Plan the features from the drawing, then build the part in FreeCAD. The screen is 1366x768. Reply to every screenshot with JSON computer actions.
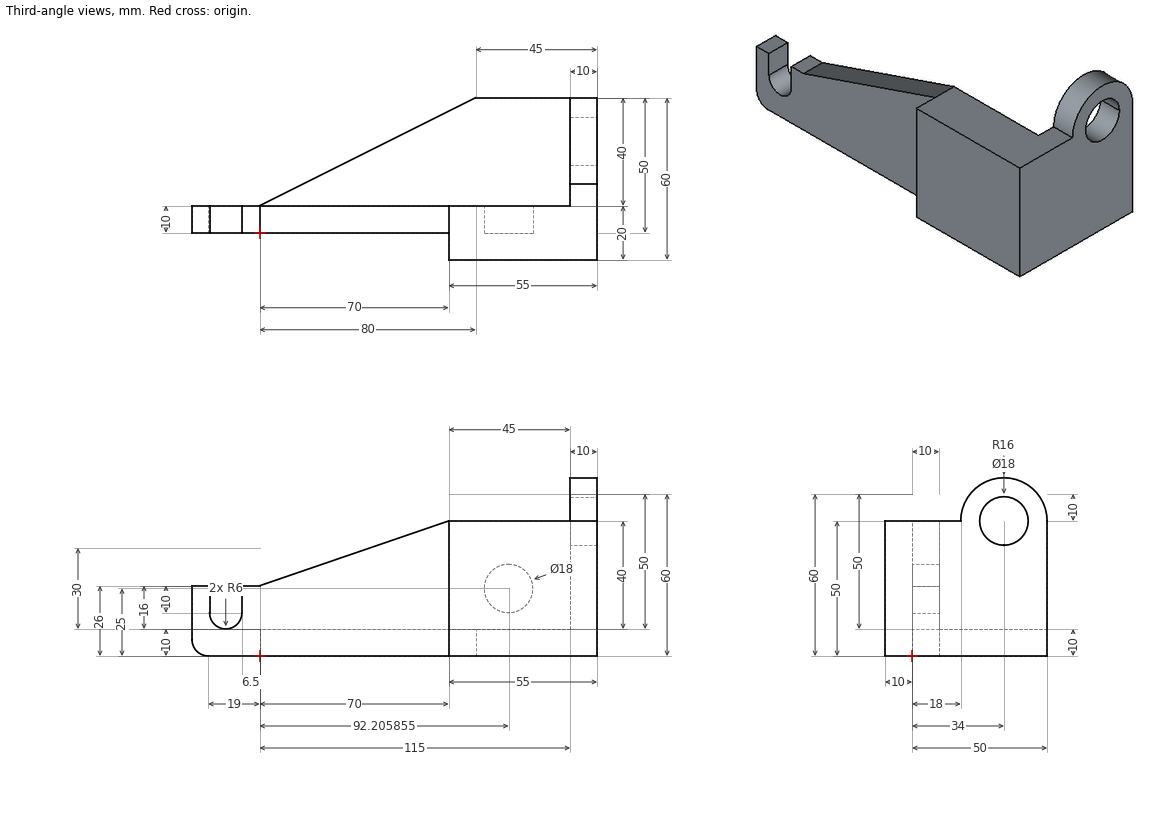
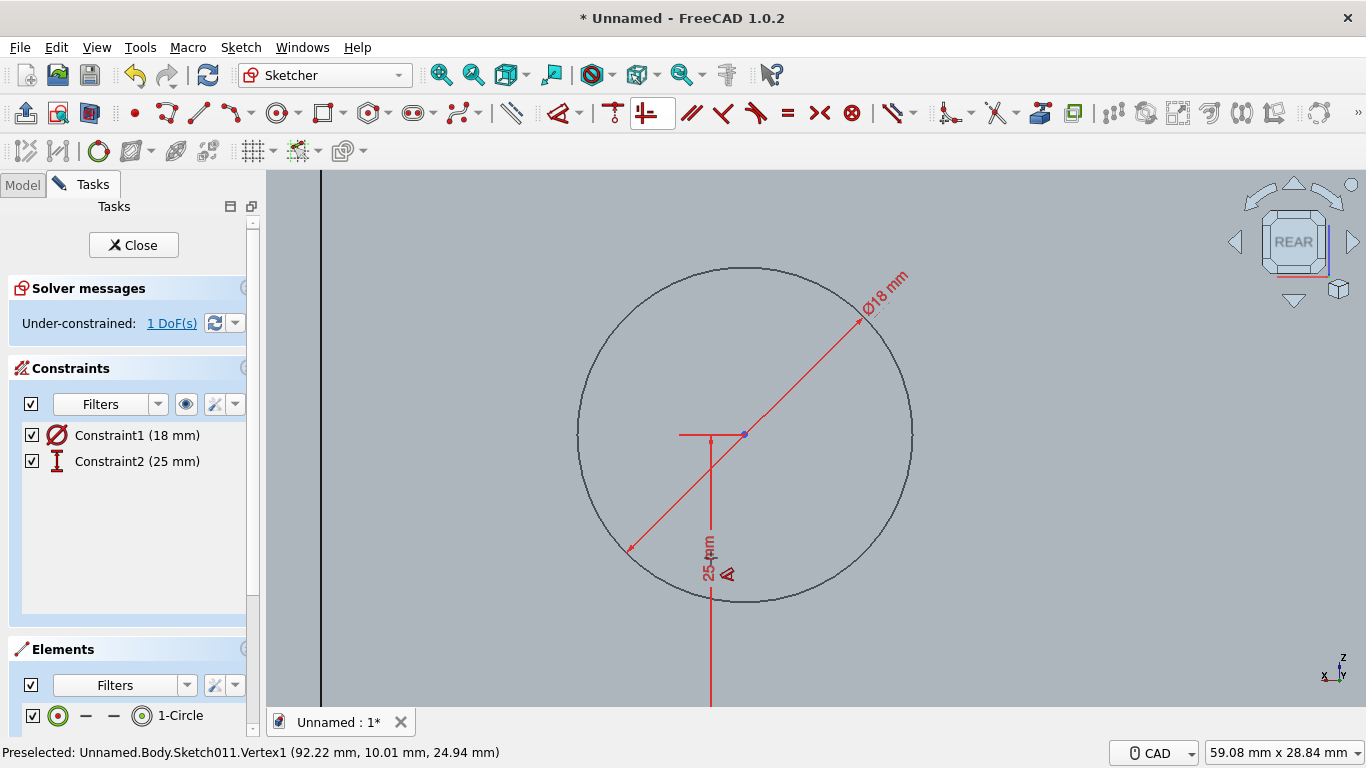
{"action": "left_click", "coordinate": [745, 435]}
{"action": "left_click", "coordinate": [973, 401]}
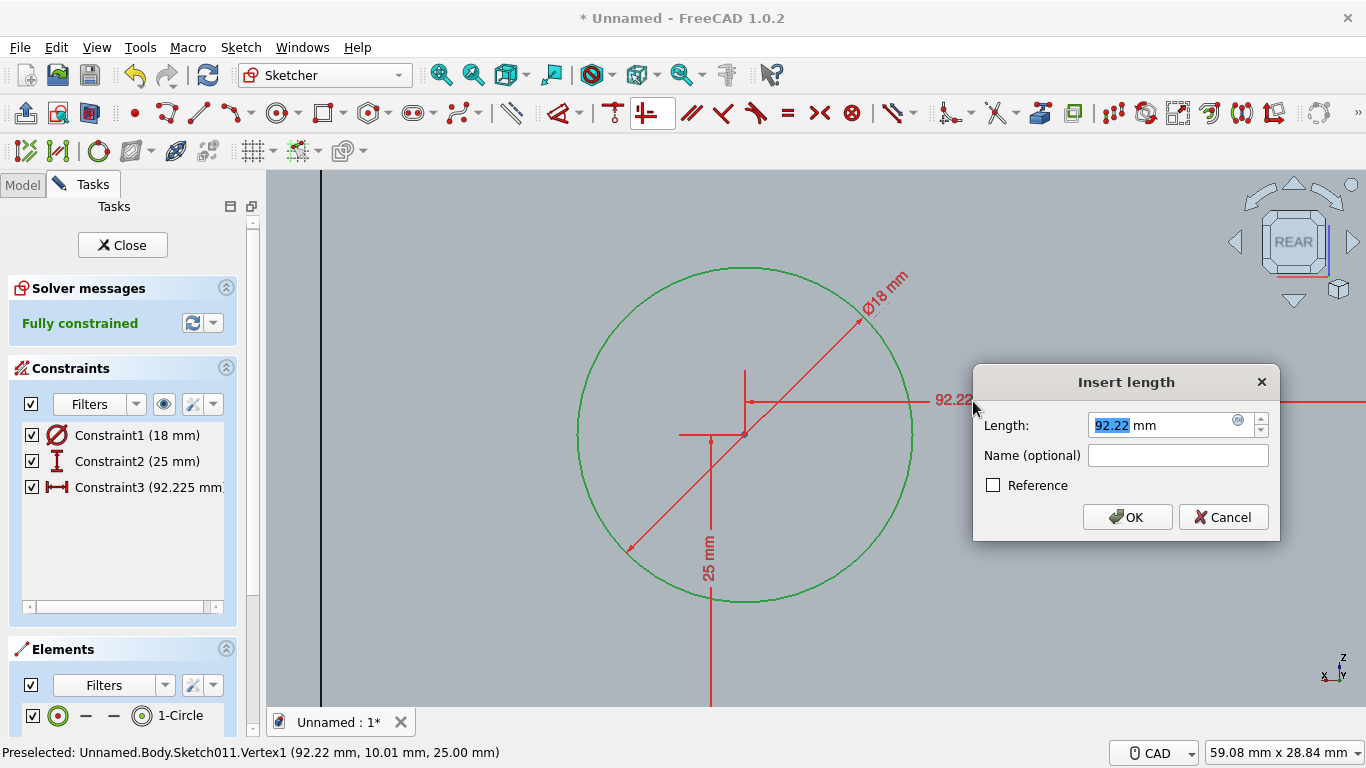
{"action": "type", "text": "92.205855"}
{"action": "key", "text": "Return"}
{"action": "key", "text": "Escape"}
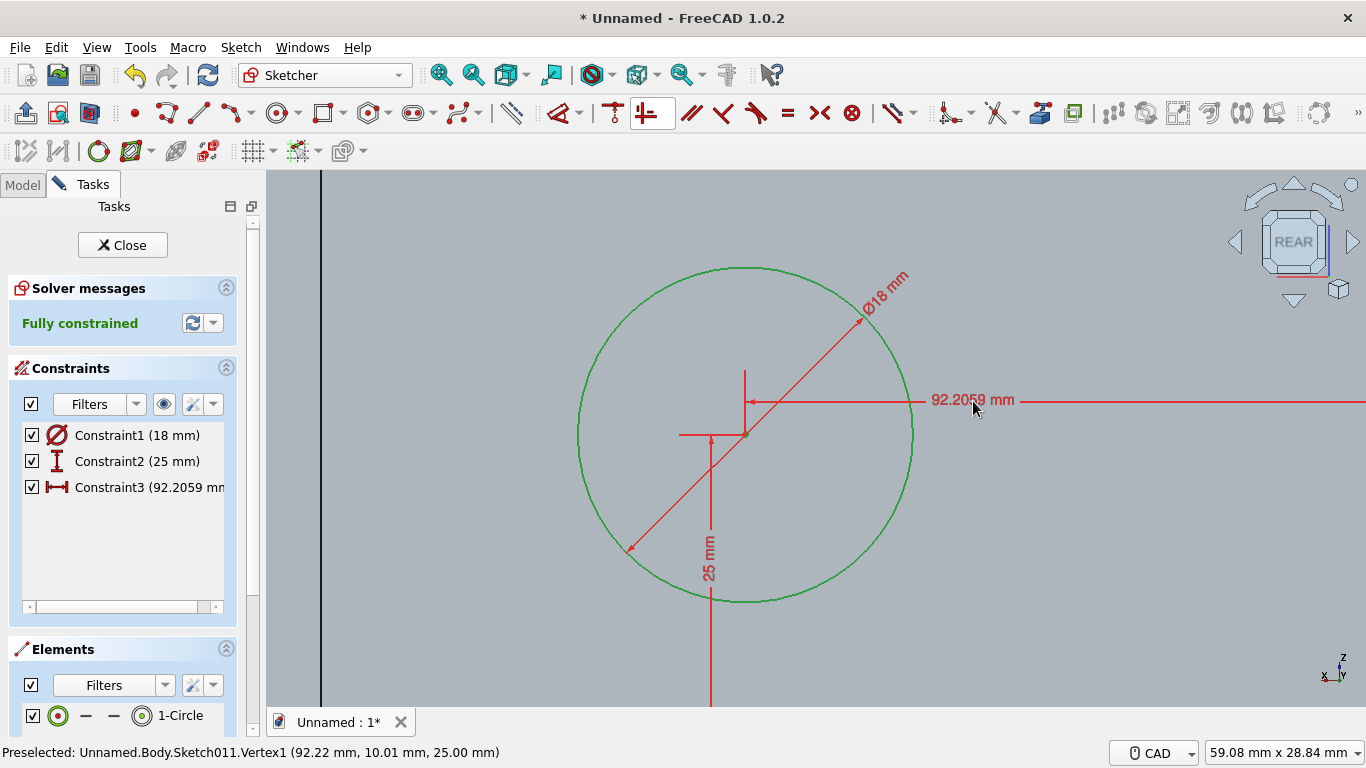
{"action": "left_click", "coordinate": [123, 245]}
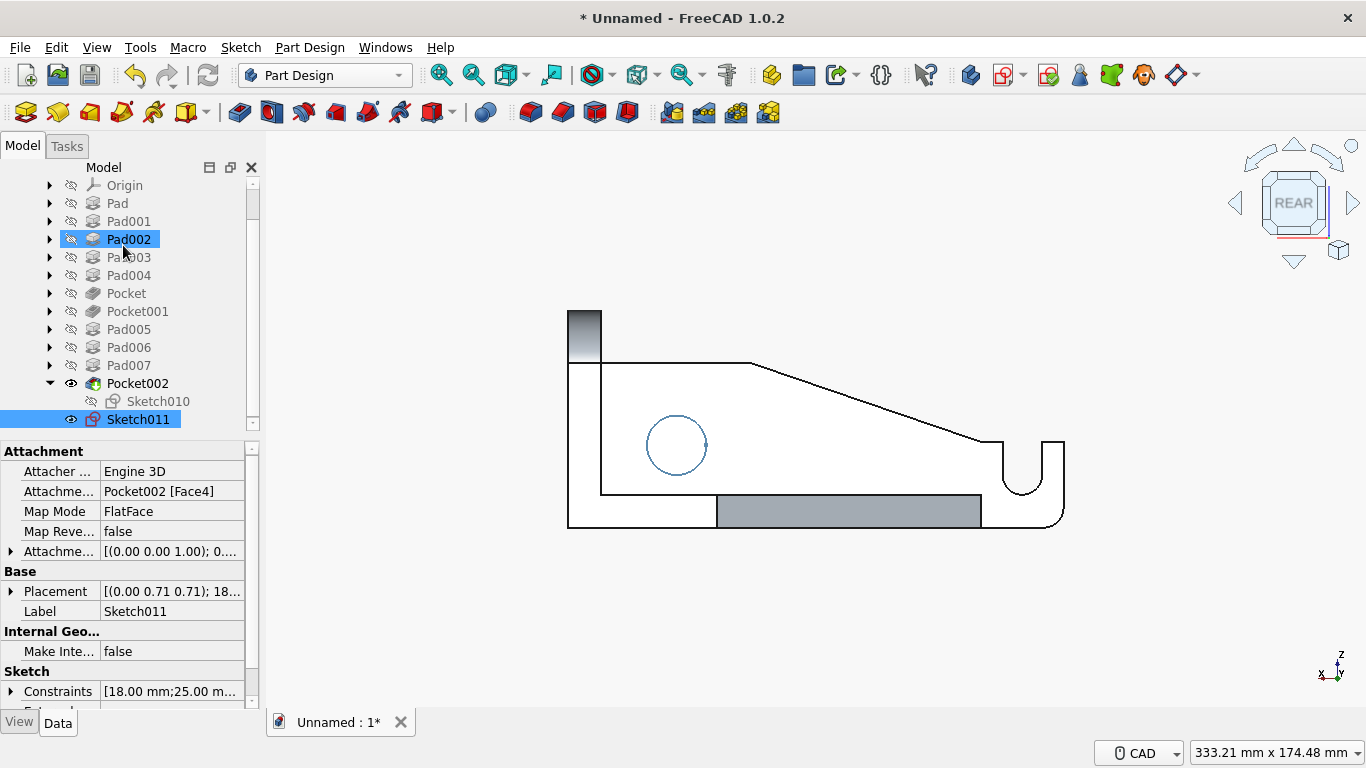
{"action": "left_click", "coordinate": [240, 112]}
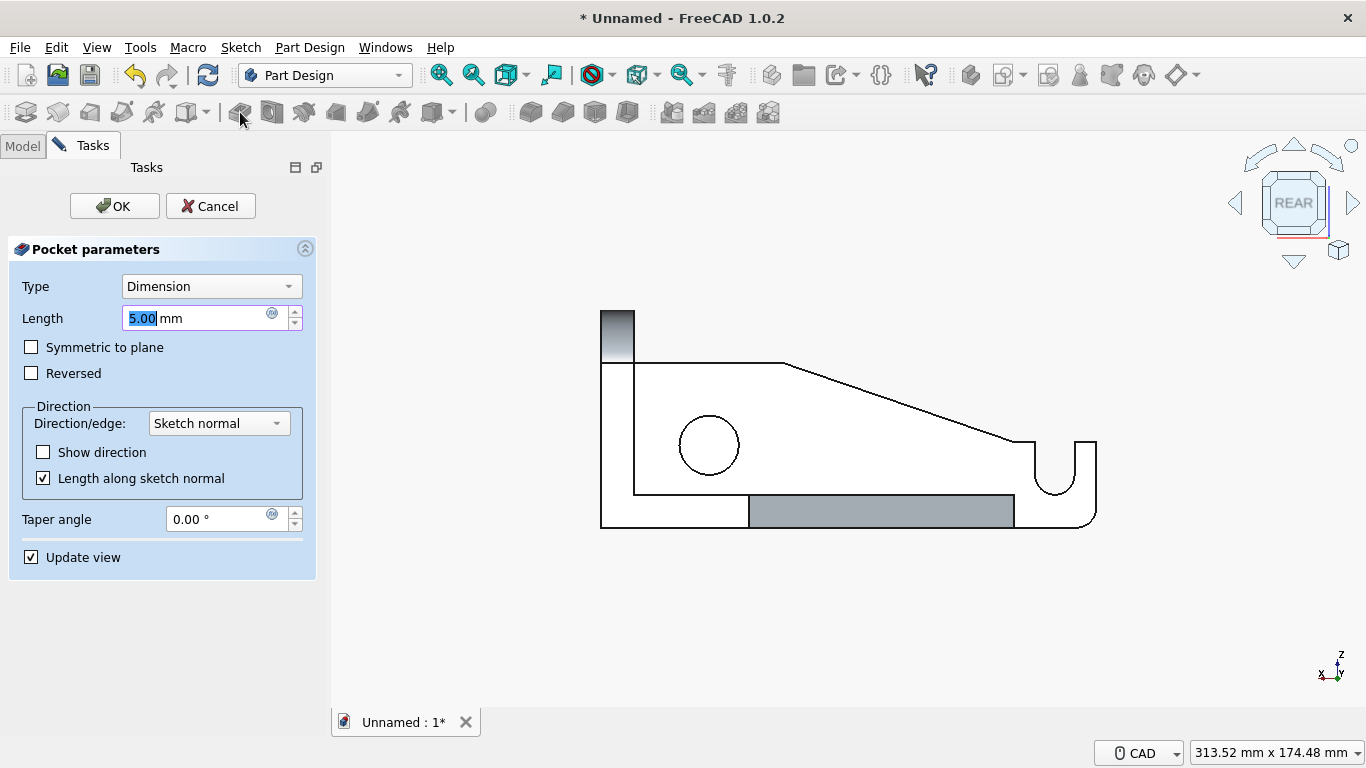
{"action": "type", "text": "10"}
{"action": "key", "text": "Tab"}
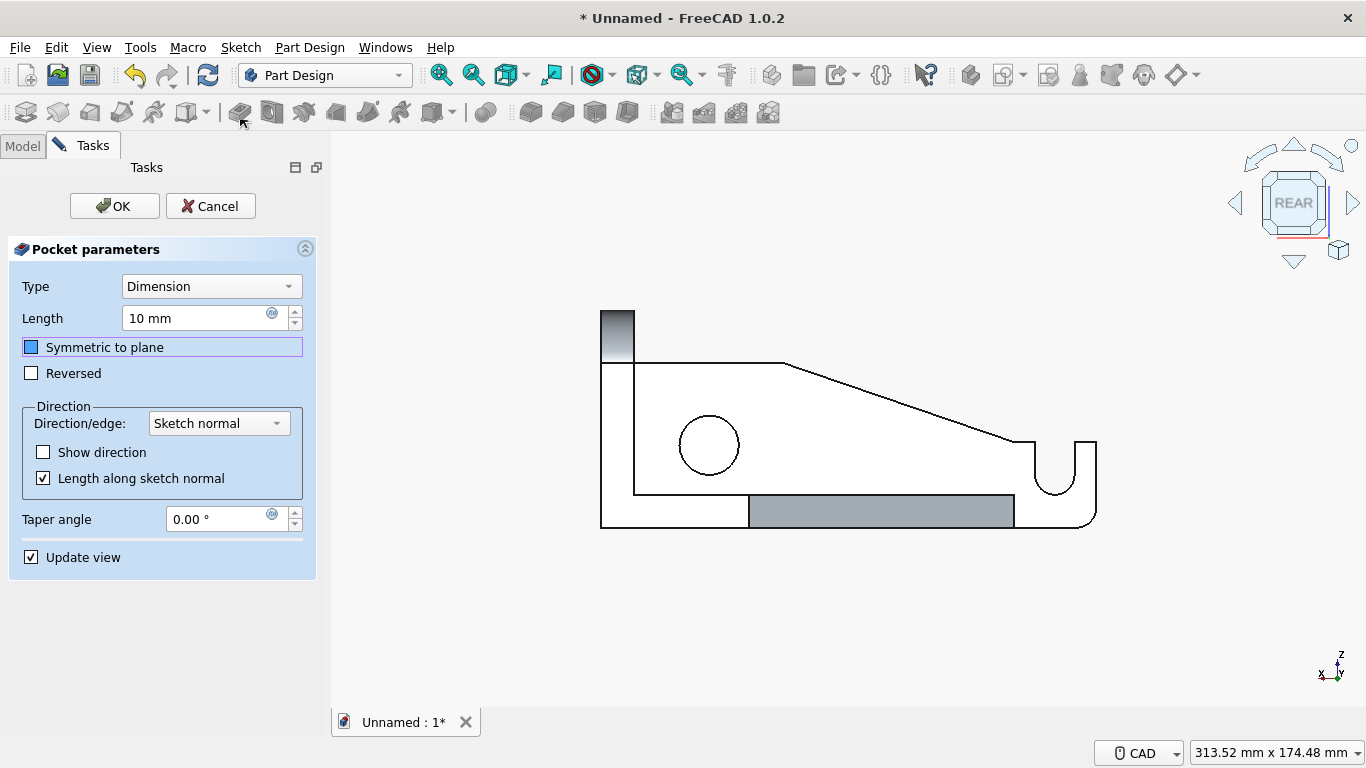
{"action": "left_click", "coordinate": [115, 206]}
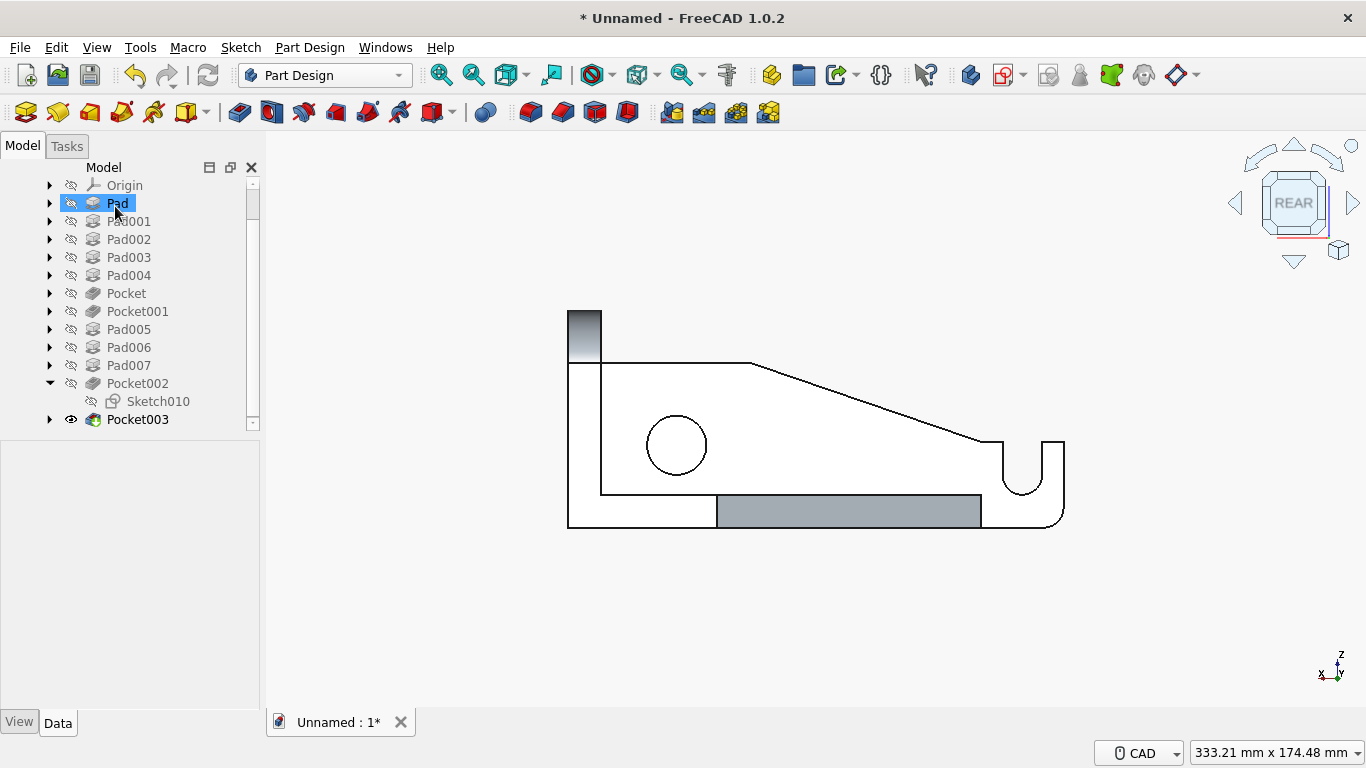
{"action": "key", "text": "0"}